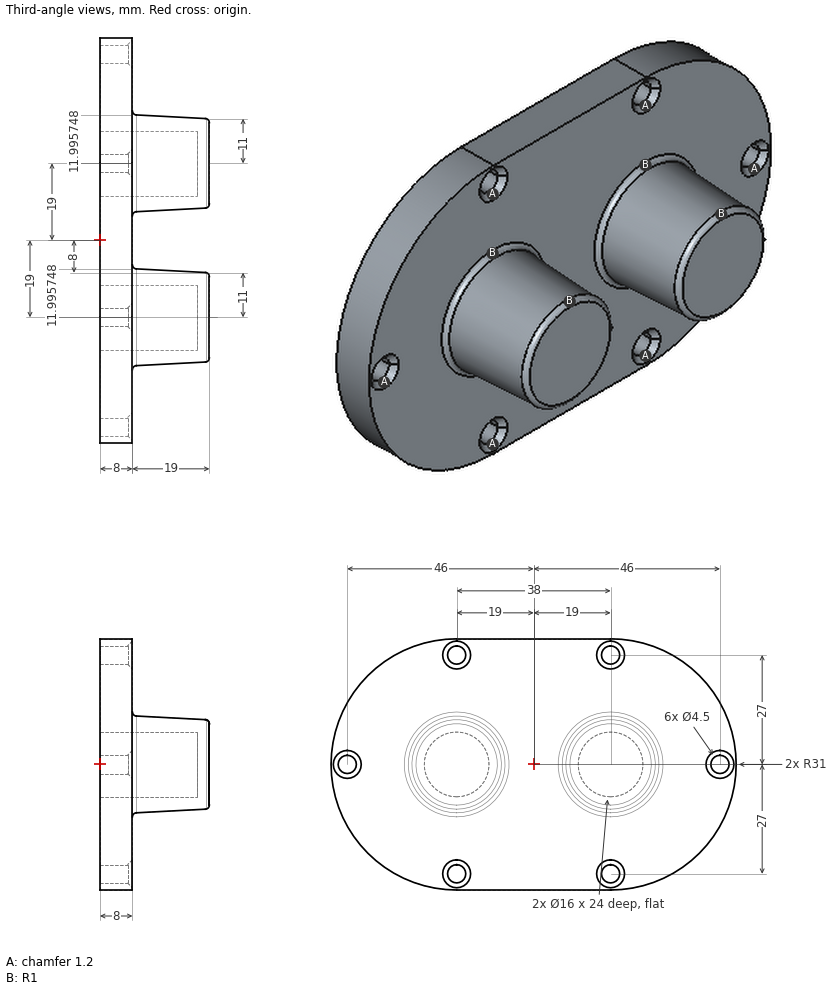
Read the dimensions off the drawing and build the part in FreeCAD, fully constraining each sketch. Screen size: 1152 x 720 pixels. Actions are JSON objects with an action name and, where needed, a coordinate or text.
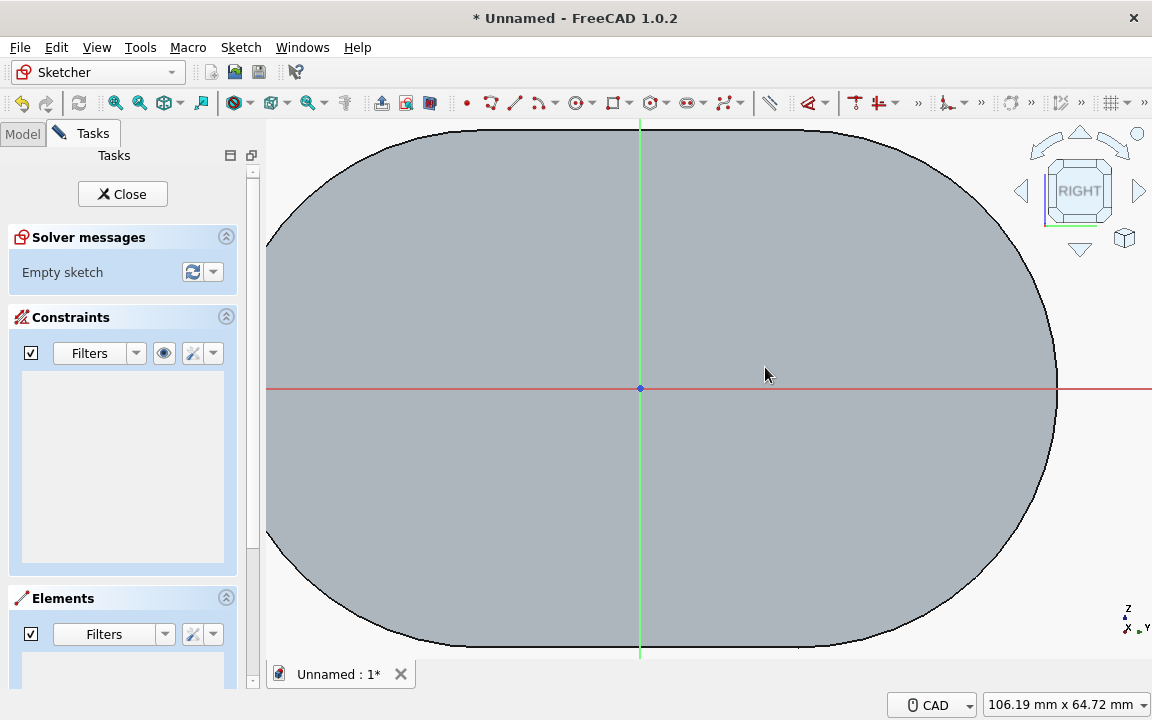
{"action": "left_click", "coordinate": [576, 104]}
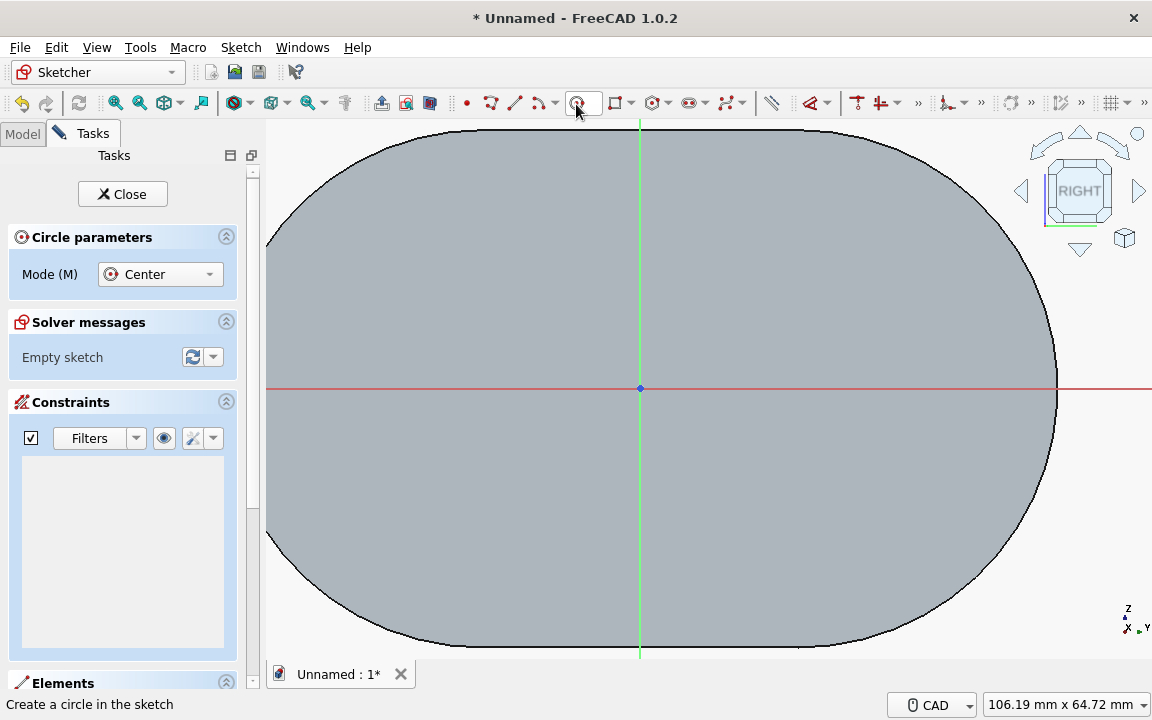
{"action": "left_click", "coordinate": [799, 389]}
{"action": "mouse_move", "coordinate": [846, 342]}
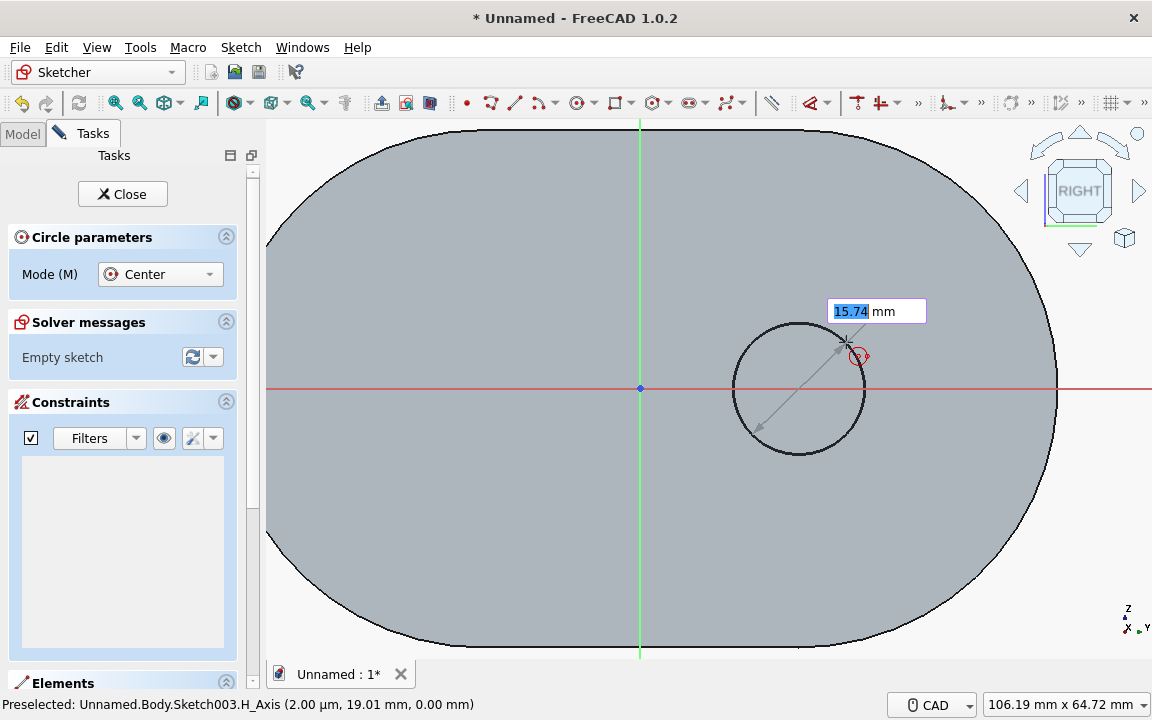
{"action": "type", "text": "16"}
{"action": "key", "text": "Return"}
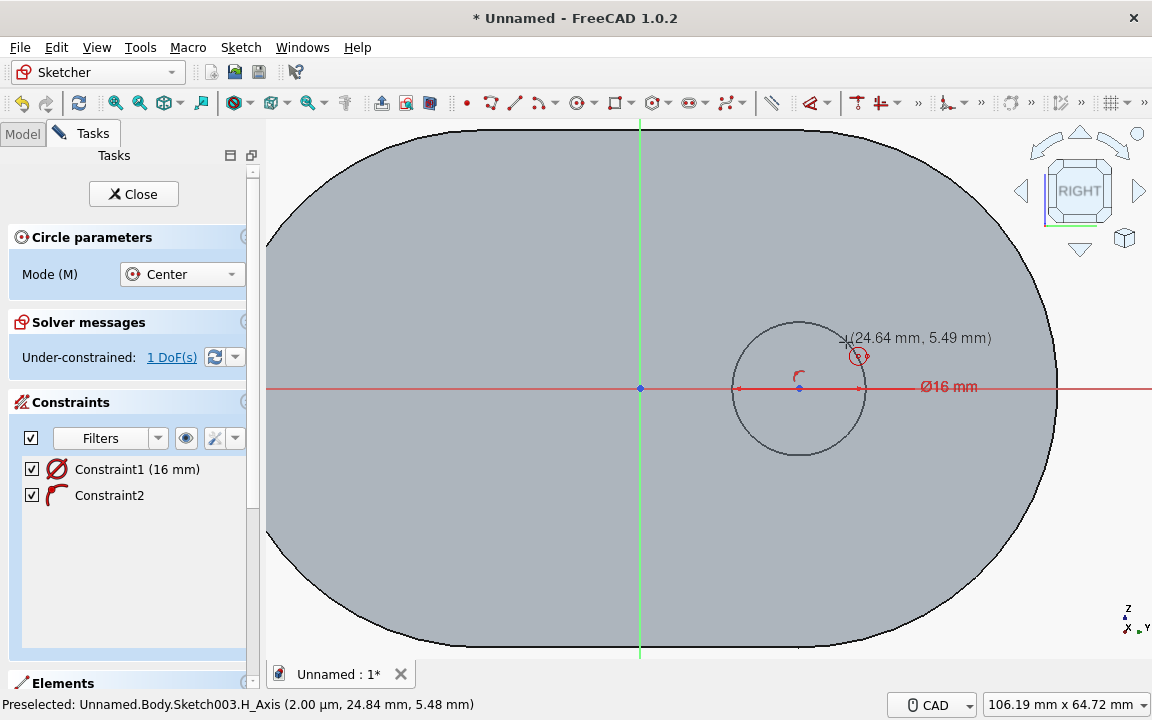
{"action": "left_click", "coordinate": [482, 389]}
{"action": "mouse_move", "coordinate": [529, 342]}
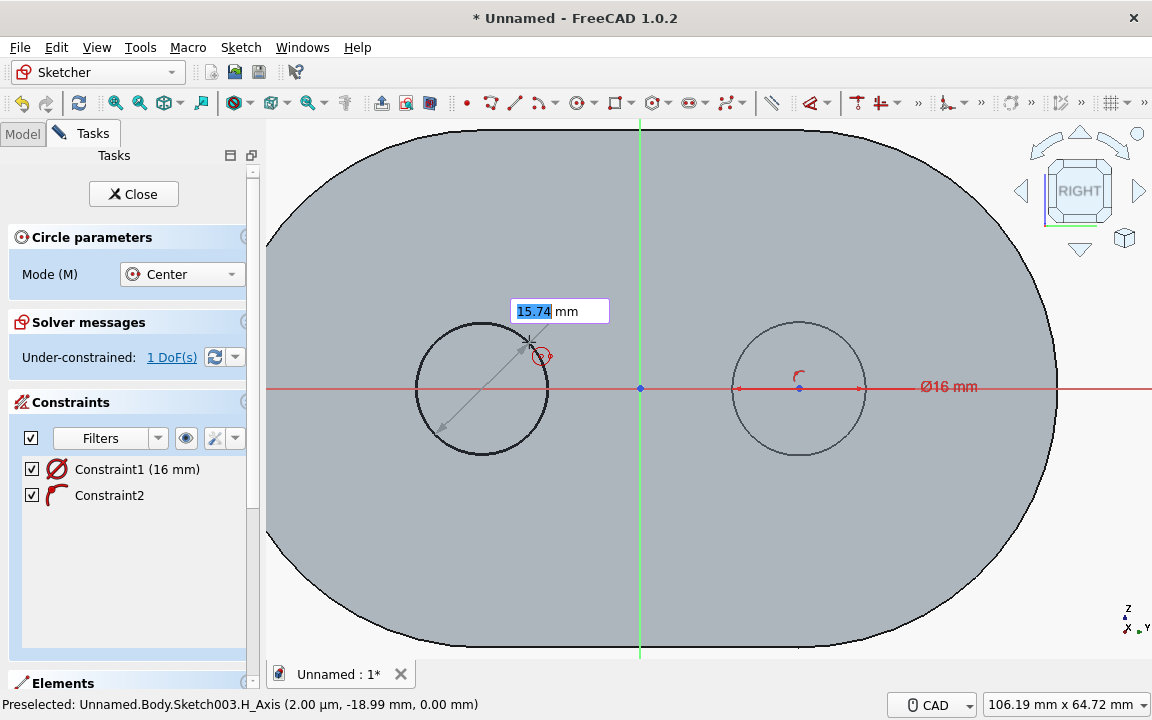
{"action": "type", "text": "16"}
{"action": "key", "text": "Return"}
{"action": "key", "text": "Escape"}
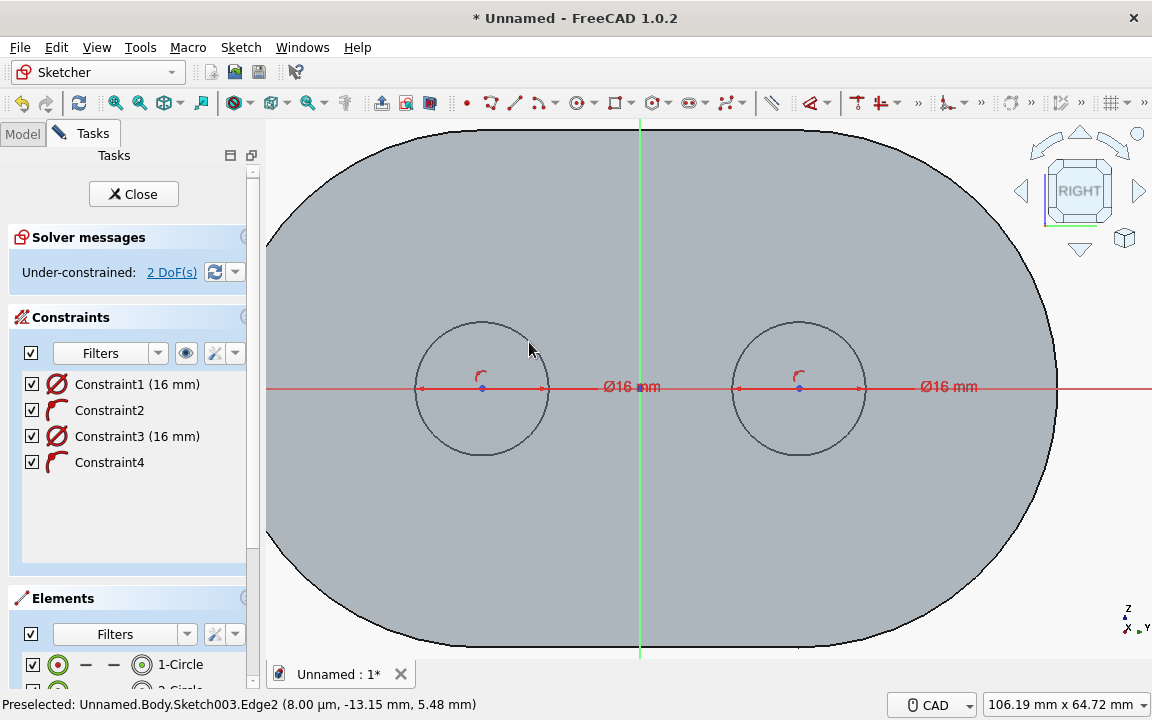
{"action": "left_click", "coordinate": [810, 104]}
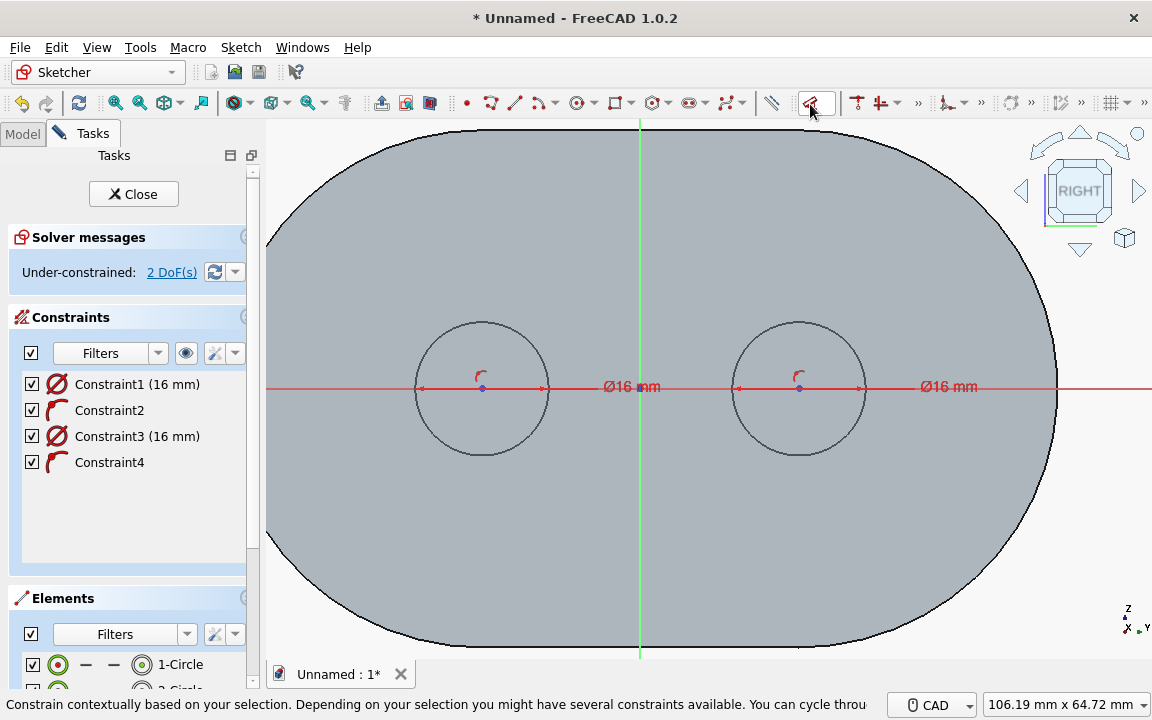
{"action": "left_click", "coordinate": [799, 389]}
{"action": "left_click", "coordinate": [720, 423]}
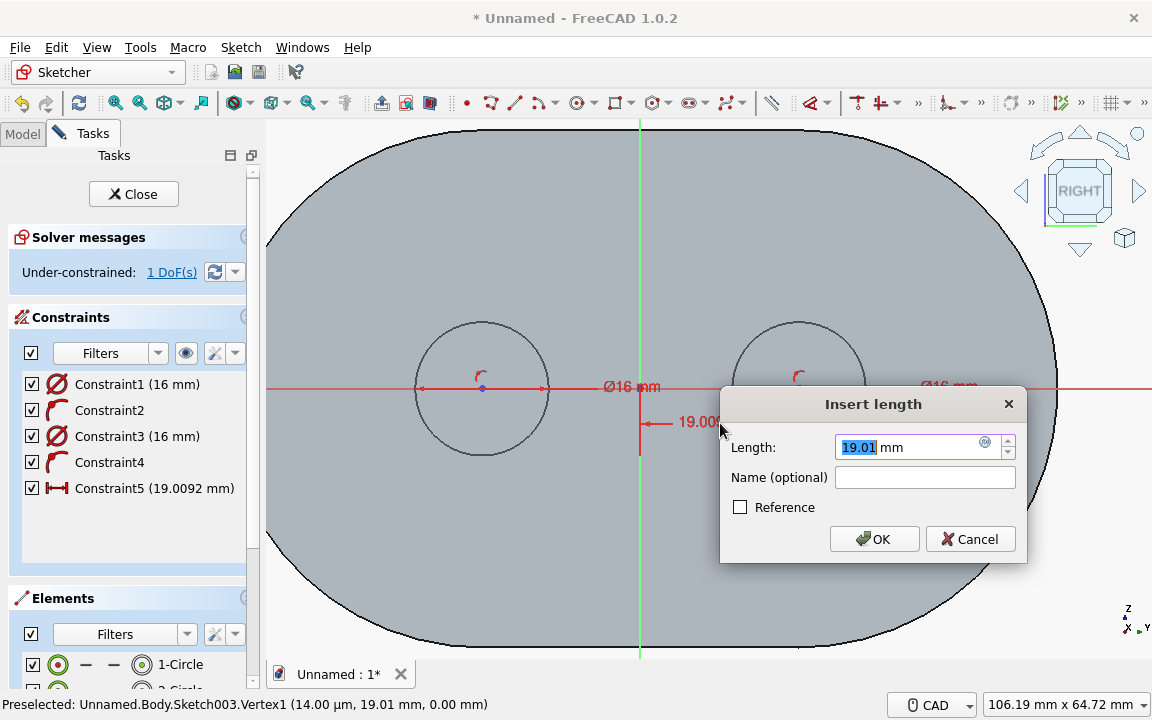
{"action": "type", "text": "19"}
{"action": "key", "text": "Return"}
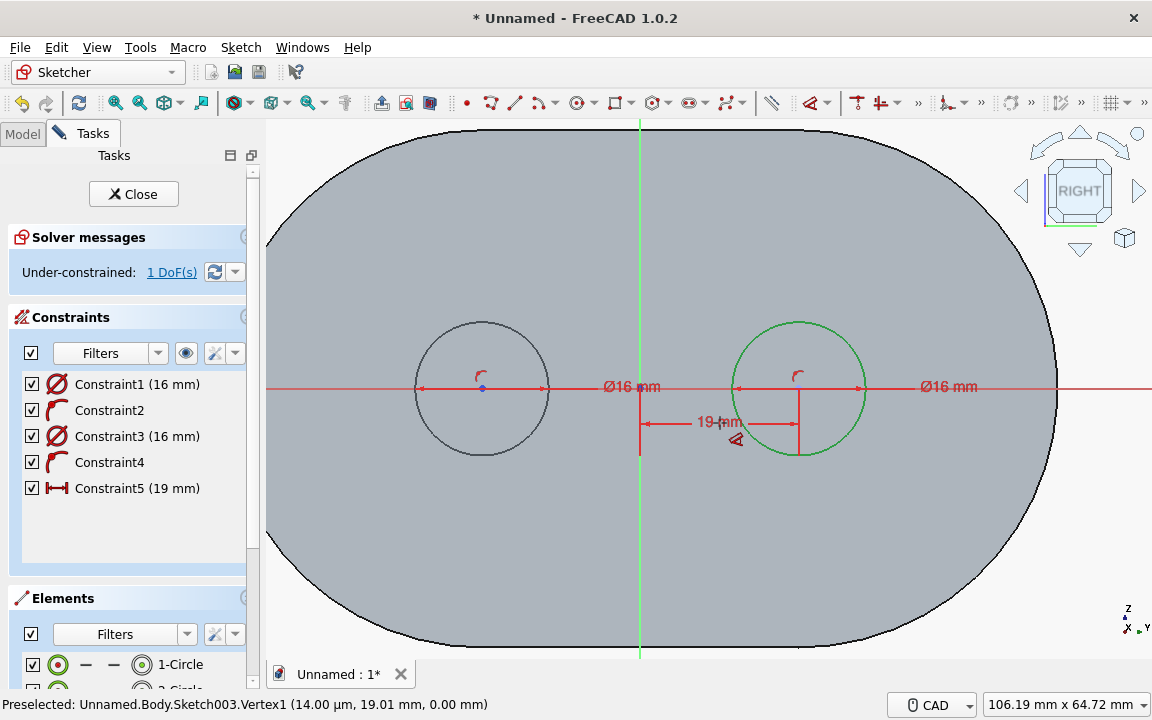
{"action": "left_click", "coordinate": [482, 389]}
{"action": "left_click", "coordinate": [561, 423]}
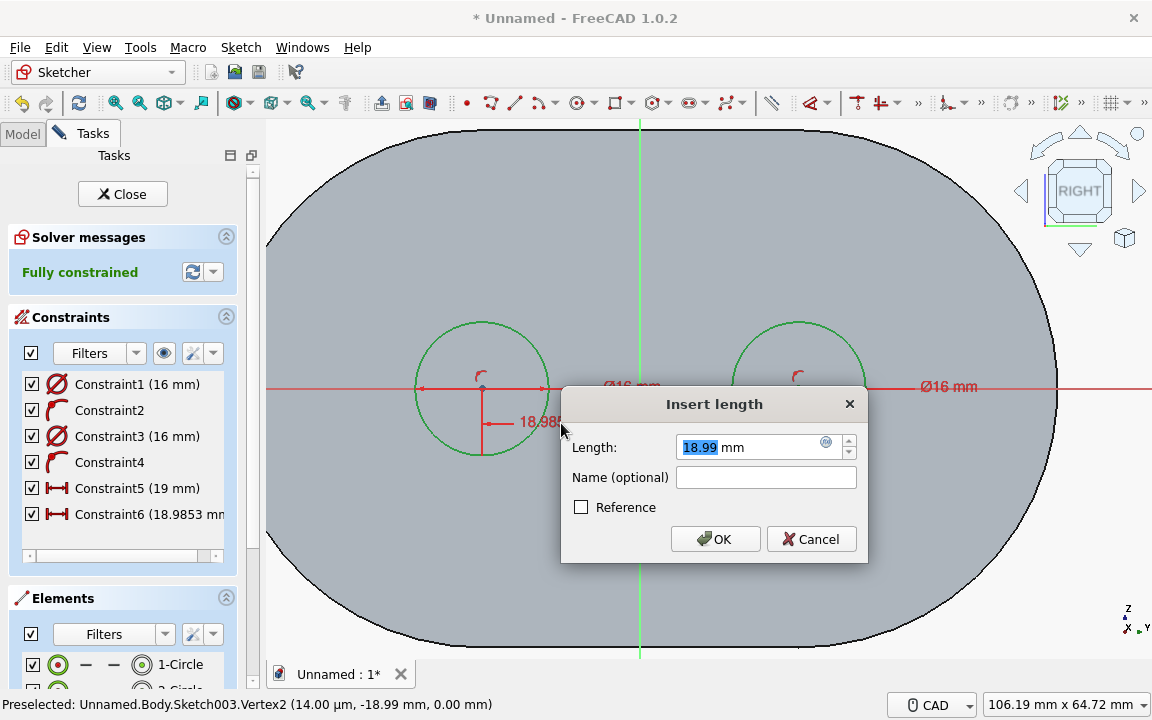
{"action": "type", "text": "19"}
{"action": "key", "text": "Return"}
{"action": "key", "text": "Escape"}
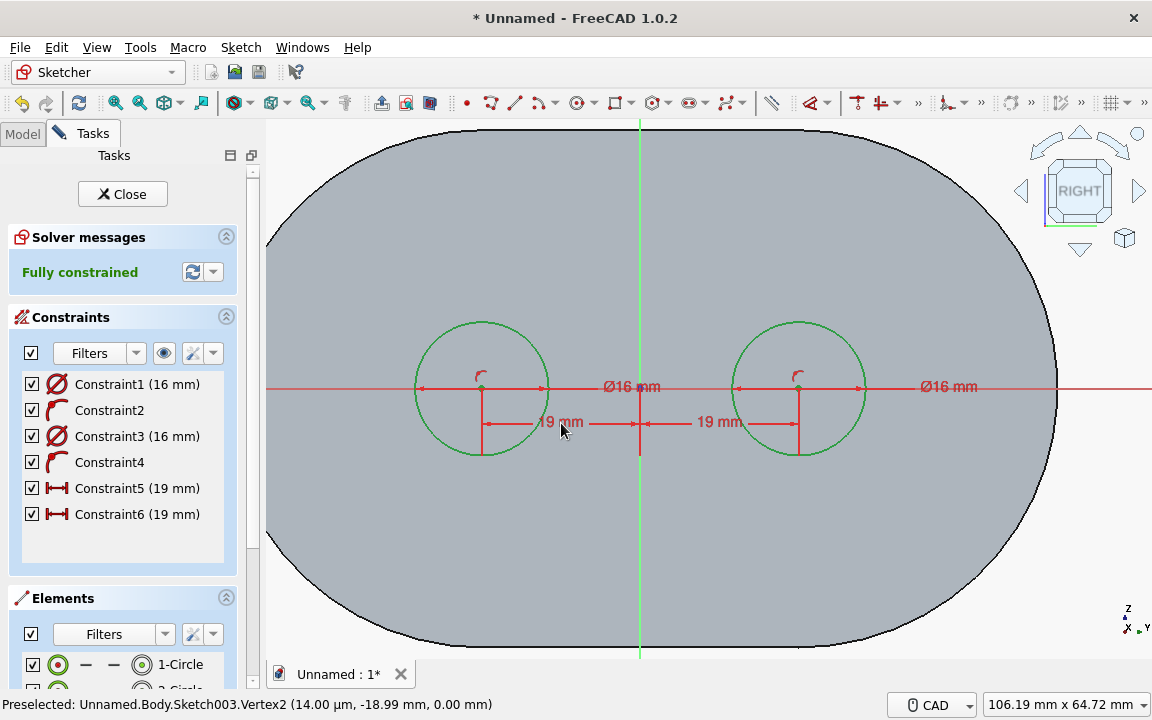
{"action": "left_click", "coordinate": [123, 194]}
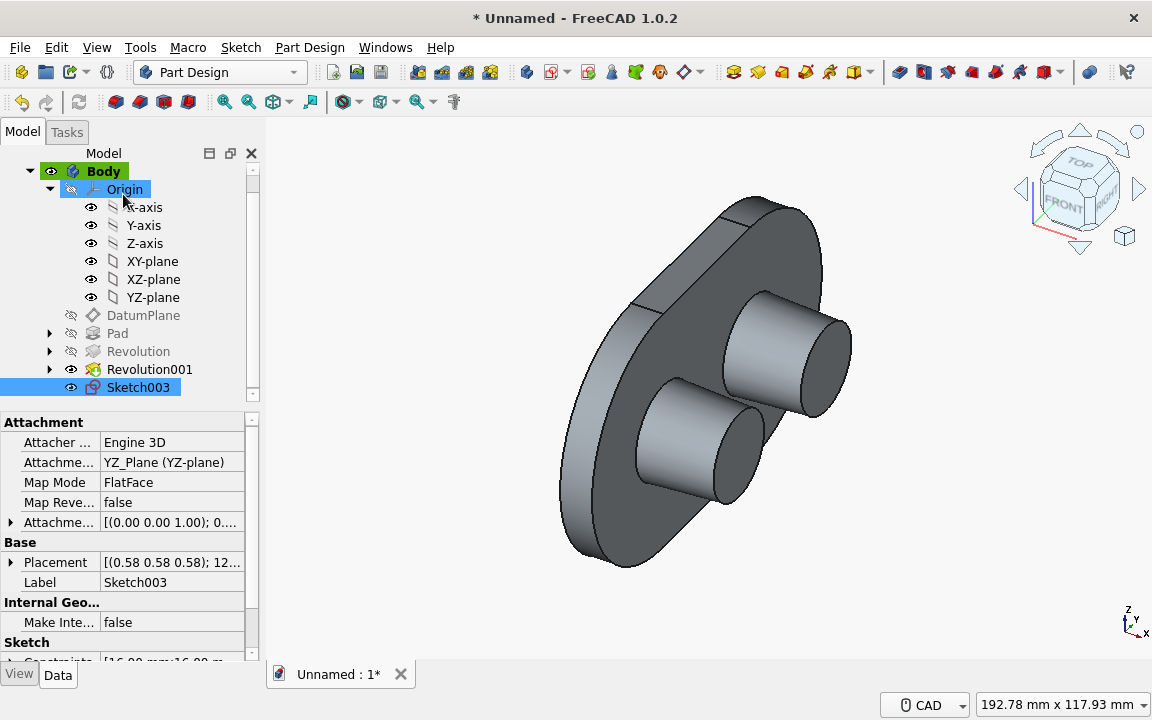
{"action": "left_click", "coordinate": [924, 72]}